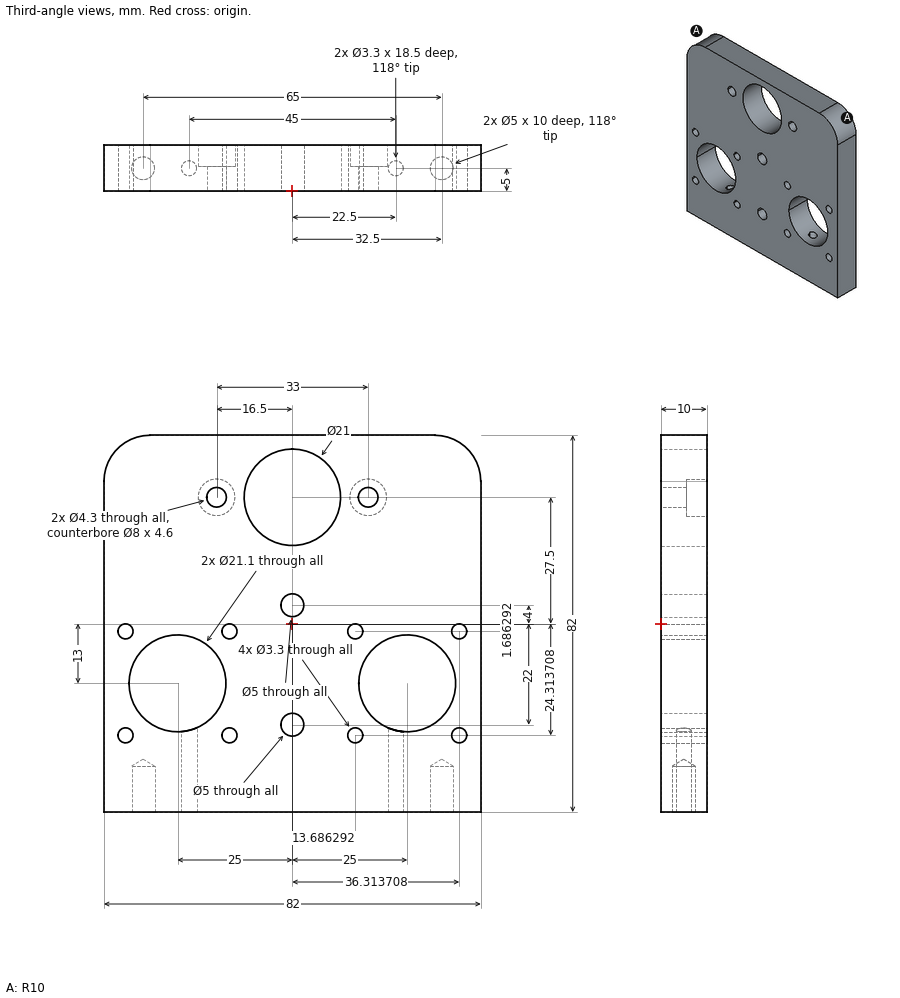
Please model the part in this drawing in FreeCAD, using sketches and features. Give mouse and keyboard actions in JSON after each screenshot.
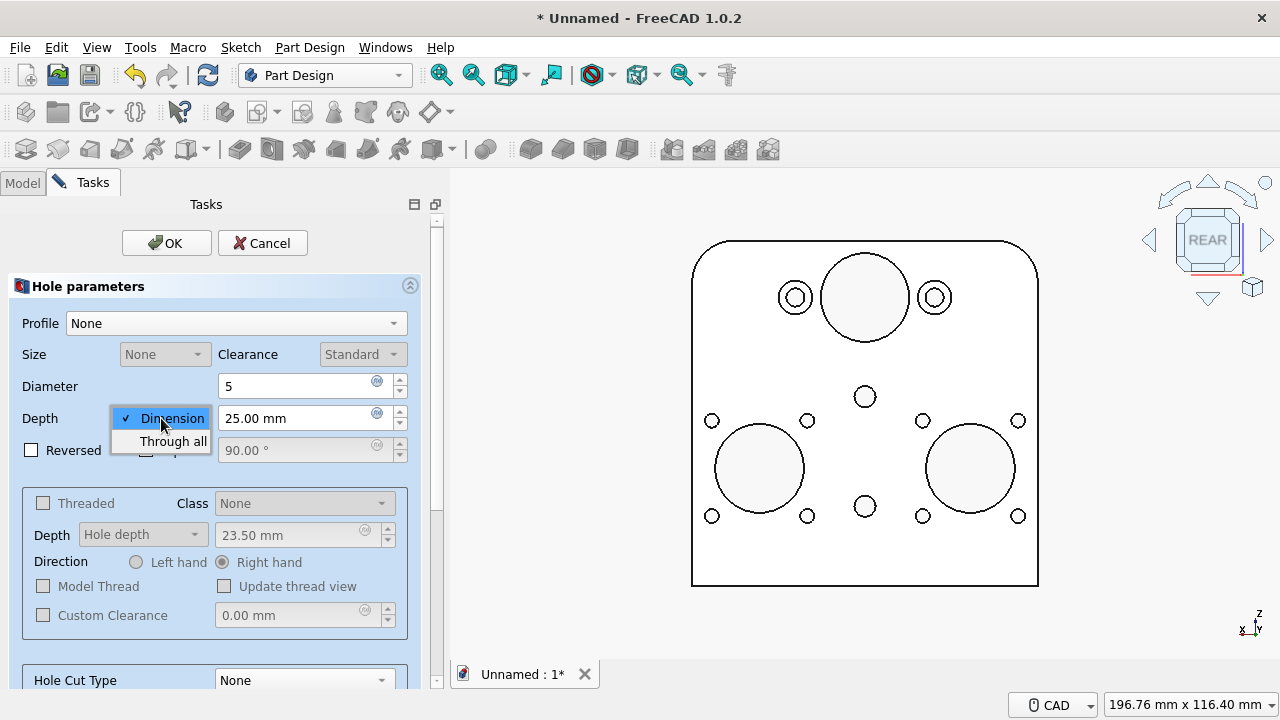
{"action": "left_click", "coordinate": [160, 442]}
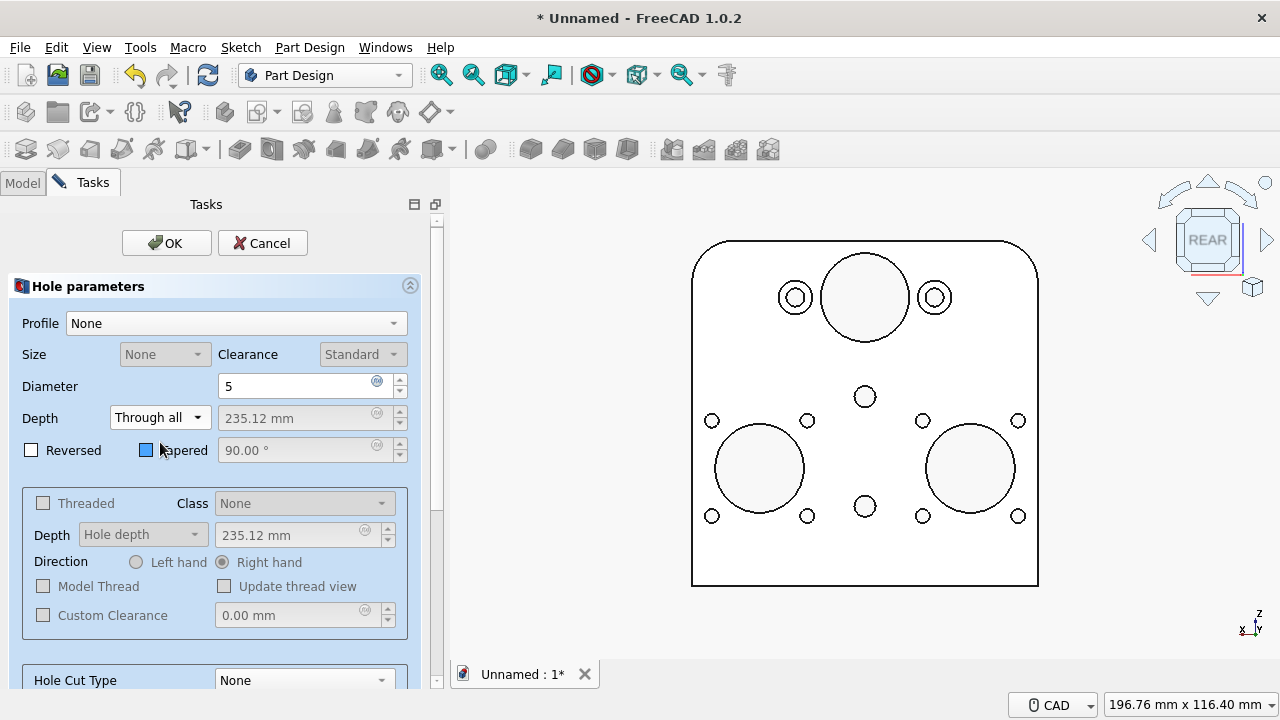
{"action": "left_click", "coordinate": [167, 243]}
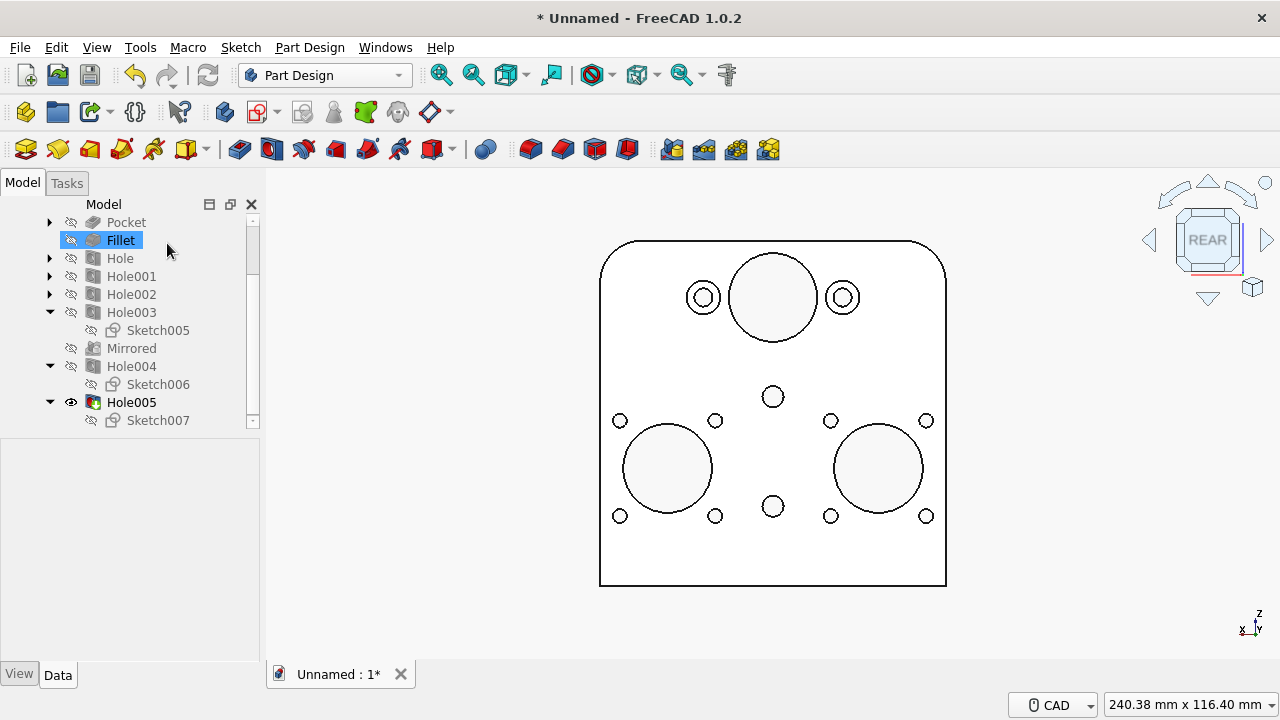
{"action": "key", "text": "5"}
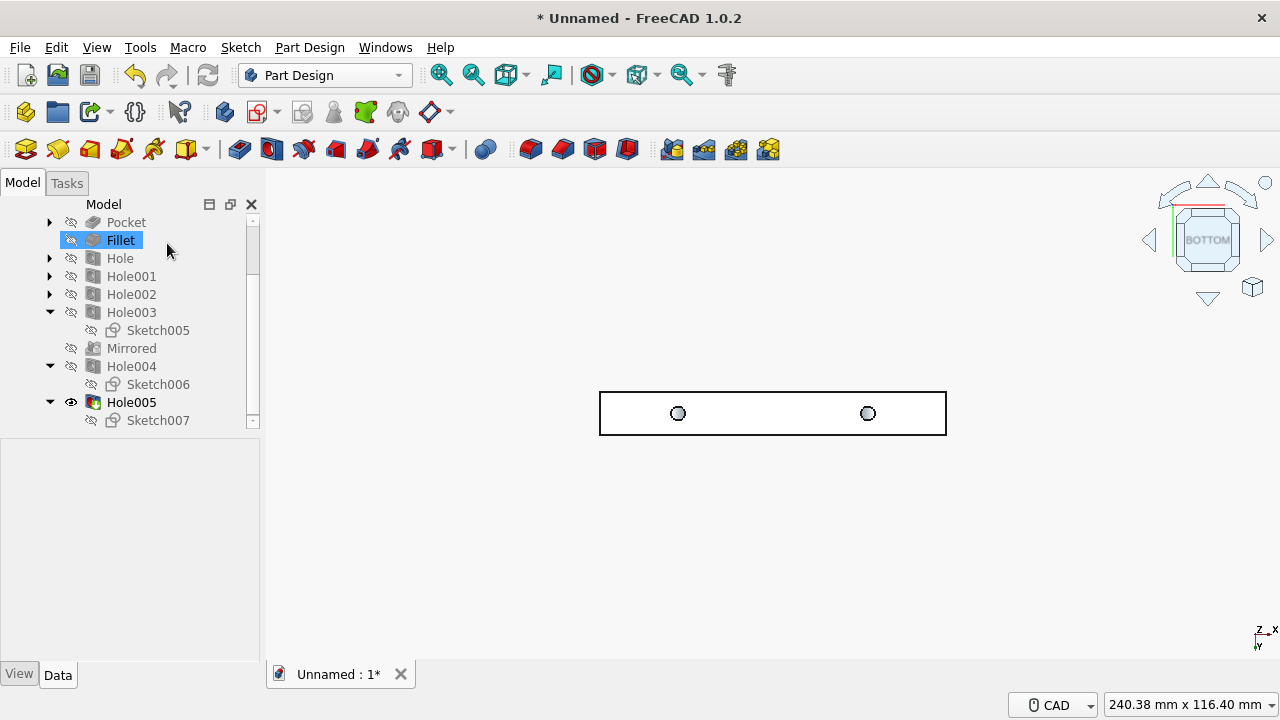
{"action": "left_click", "coordinate": [442, 76]}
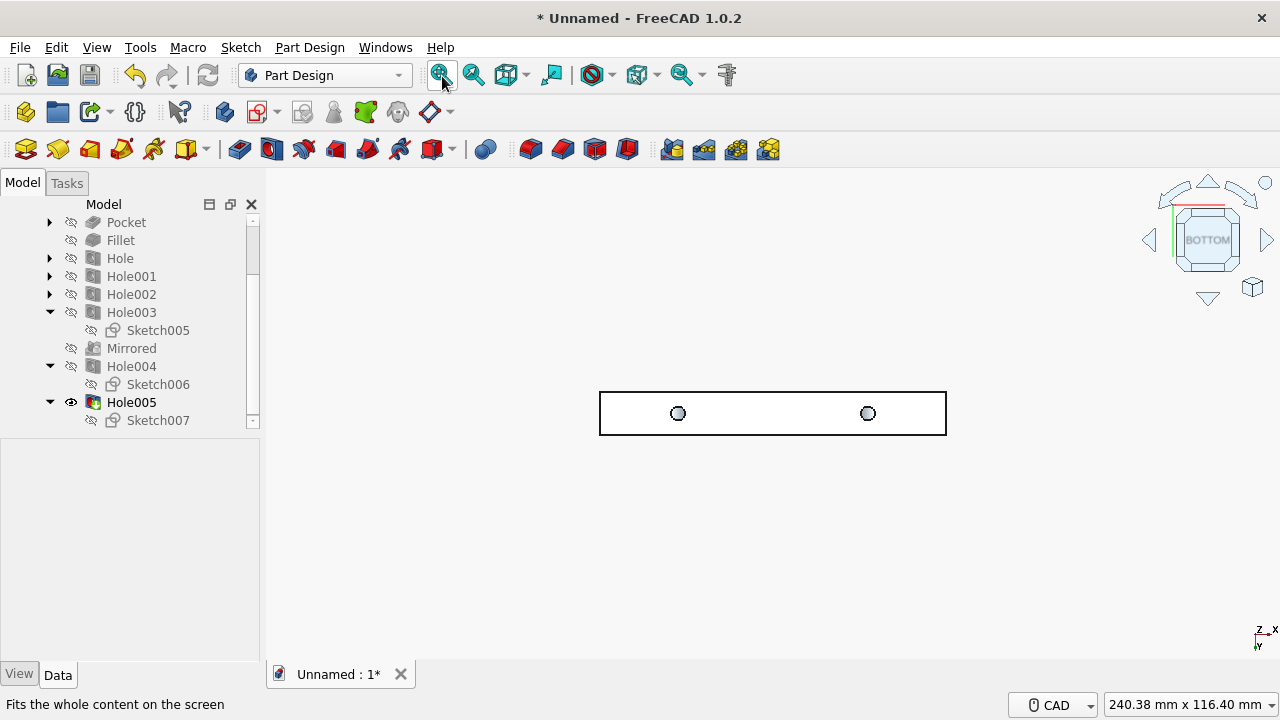
{"action": "left_click", "coordinate": [921, 412]}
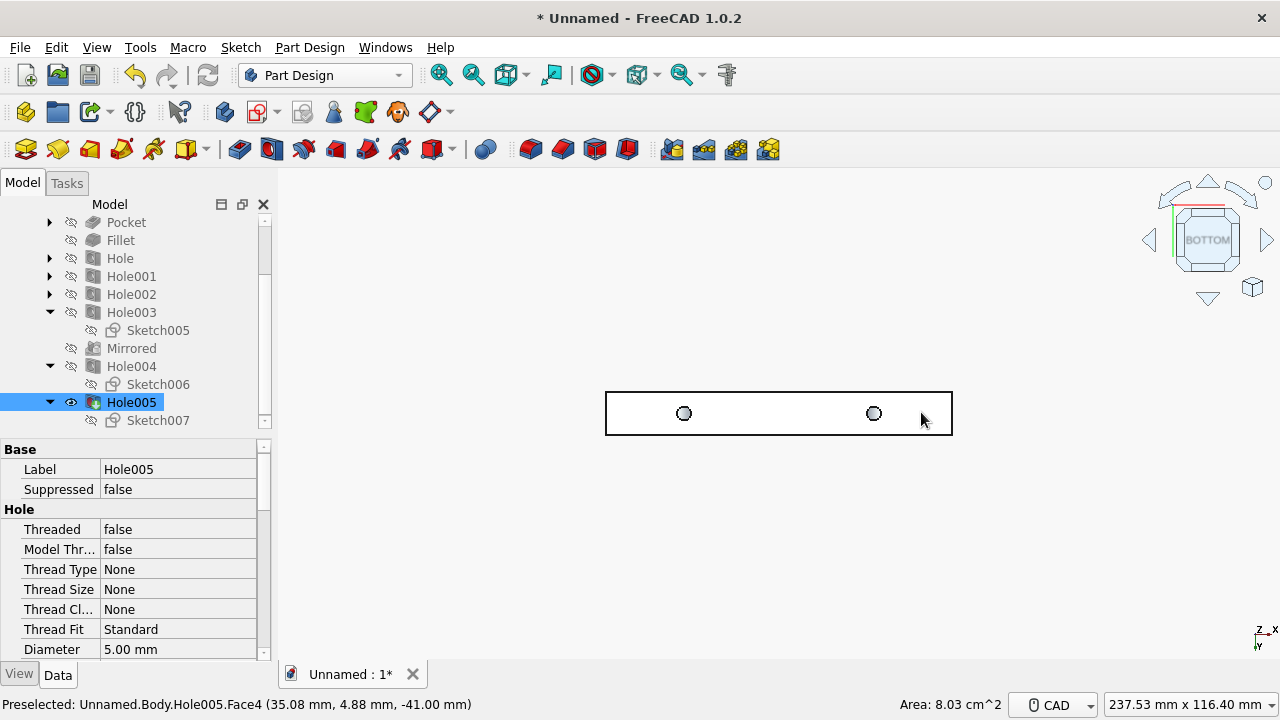
{"action": "left_click", "coordinate": [258, 112]}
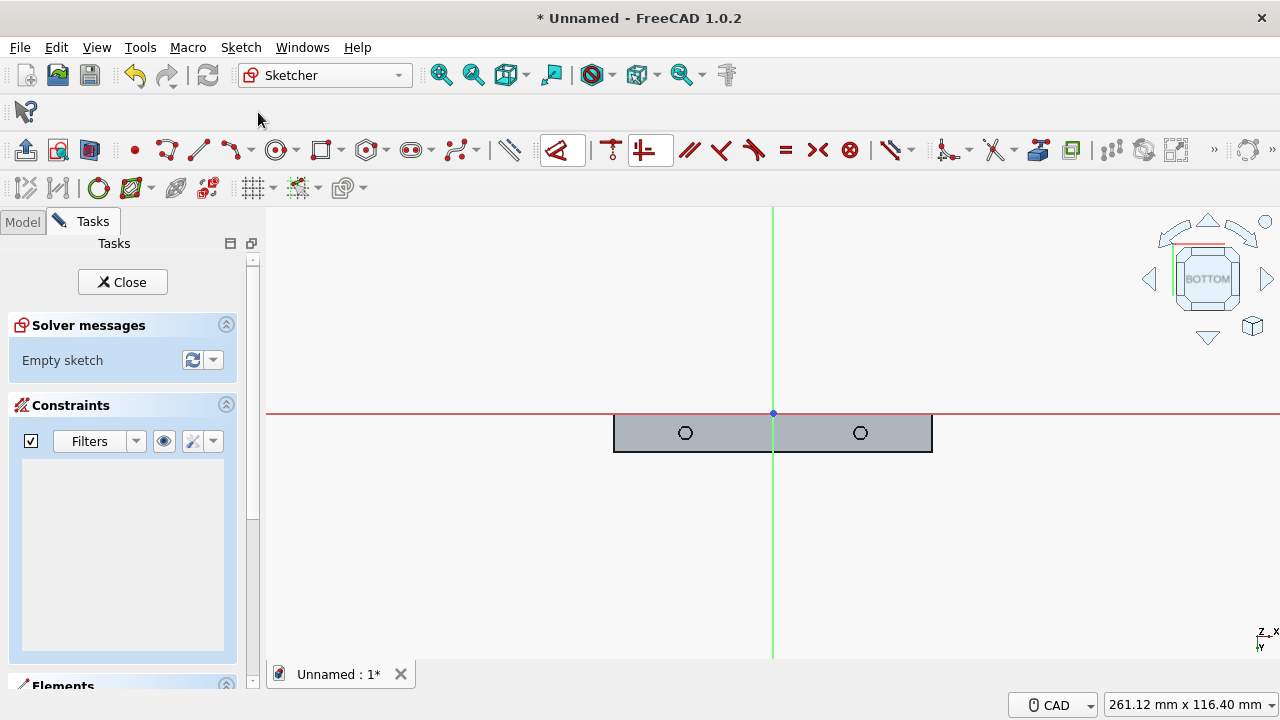
{"action": "scroll", "coordinate": [829, 424], "scroll_direction": "up", "scroll_amount": 4}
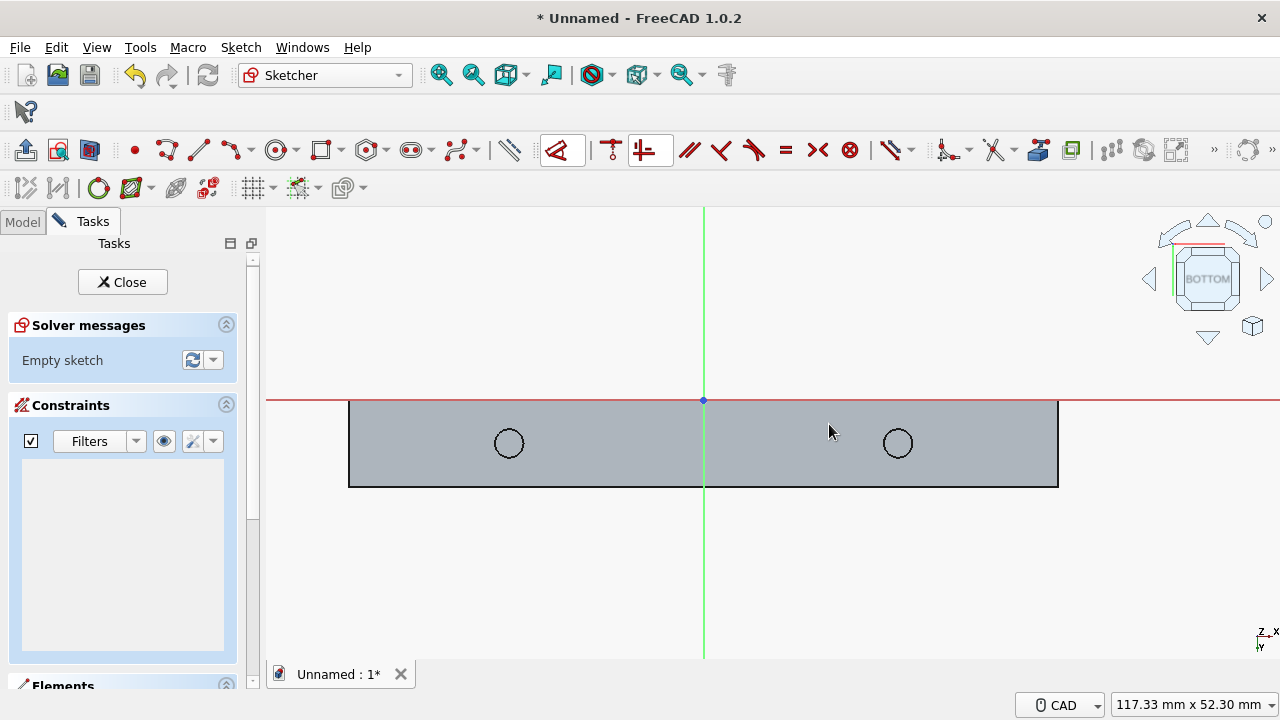
{"action": "left_click", "coordinate": [276, 150]}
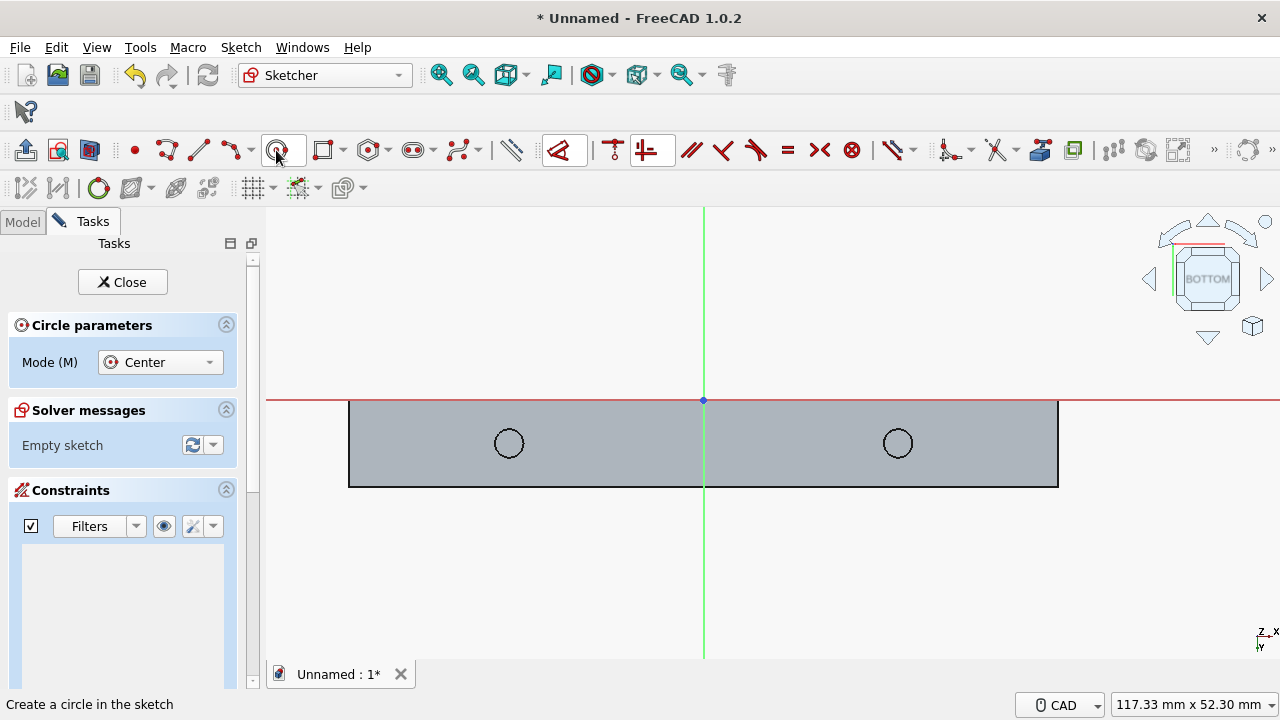
{"action": "left_click", "coordinate": [985, 443]}
{"action": "left_click", "coordinate": [1000, 428]}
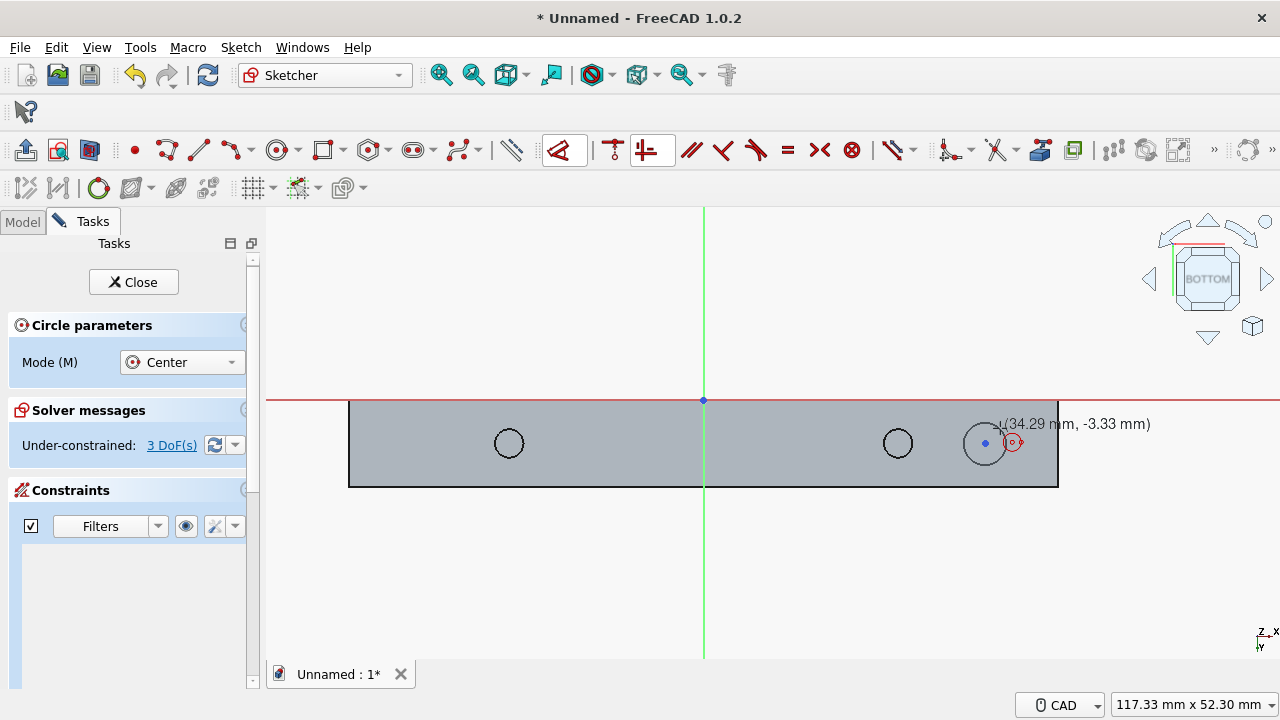
{"action": "left_click", "coordinate": [423, 443]}
{"action": "left_click", "coordinate": [438, 428]}
{"action": "key", "text": "Escape"}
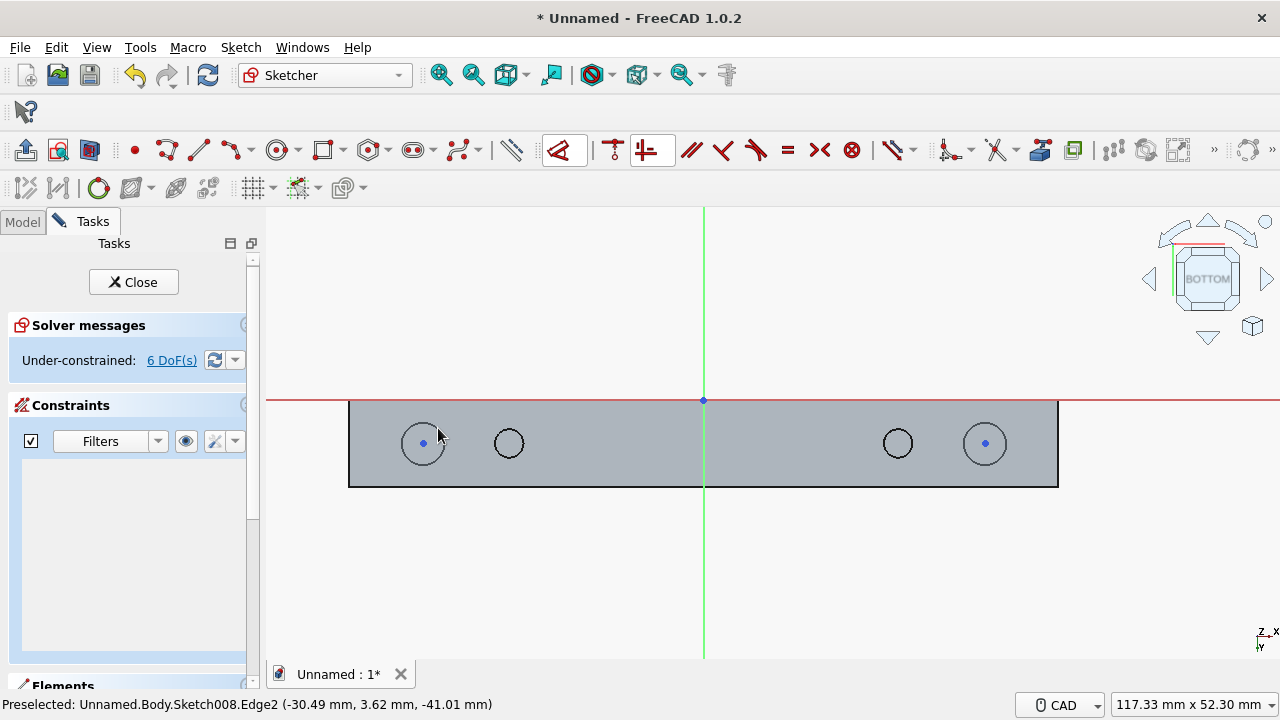
{"action": "left_click", "coordinate": [1000, 429]}